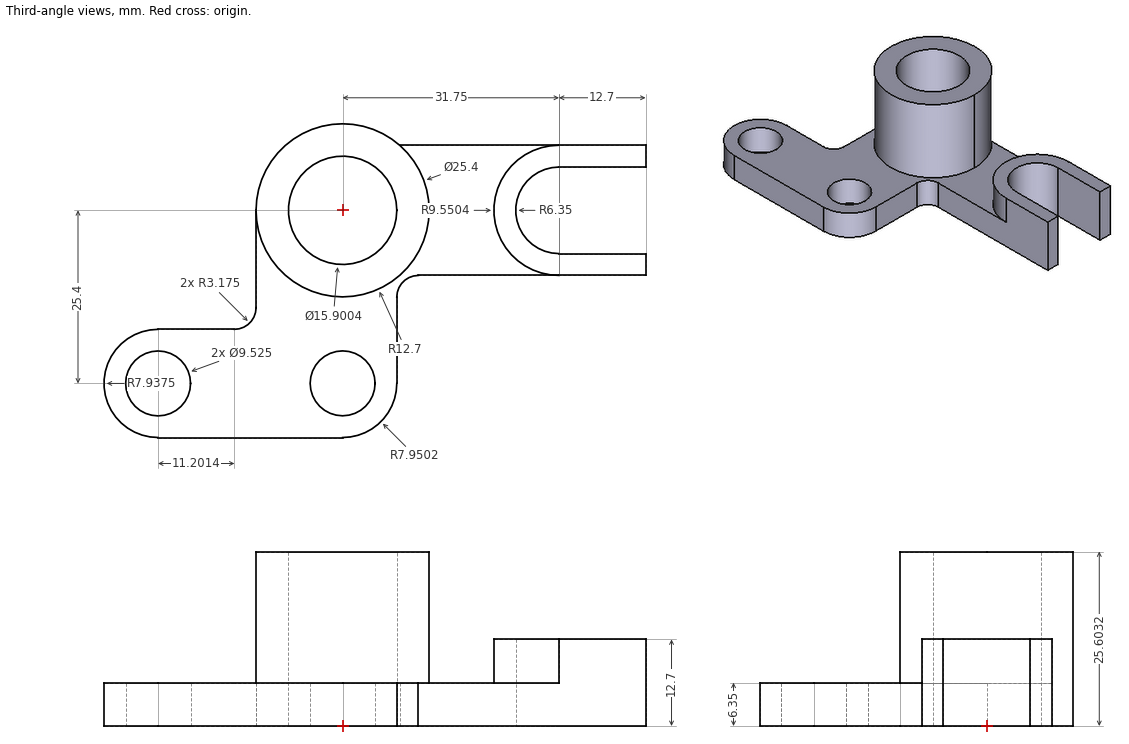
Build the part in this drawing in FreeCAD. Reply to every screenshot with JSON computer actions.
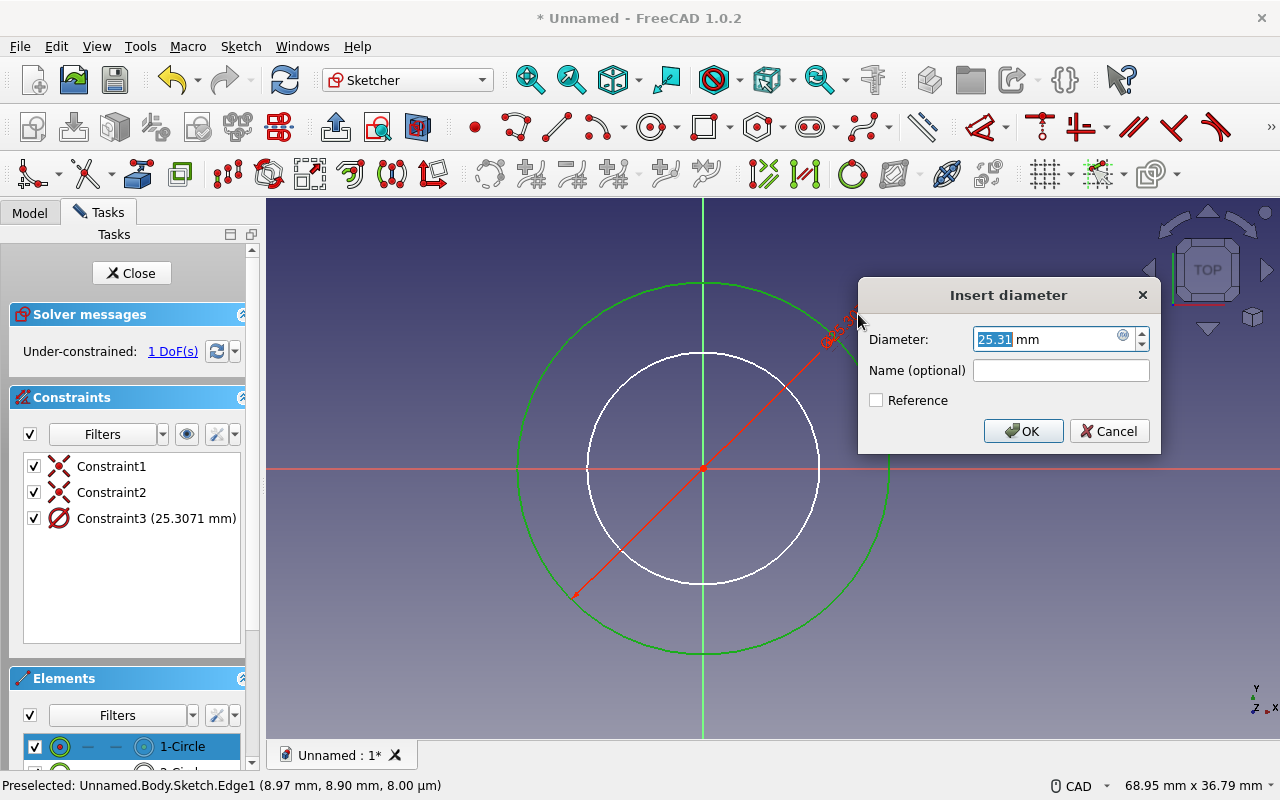
{"action": "type", "text": "25.4"}
{"action": "key", "text": "Return"}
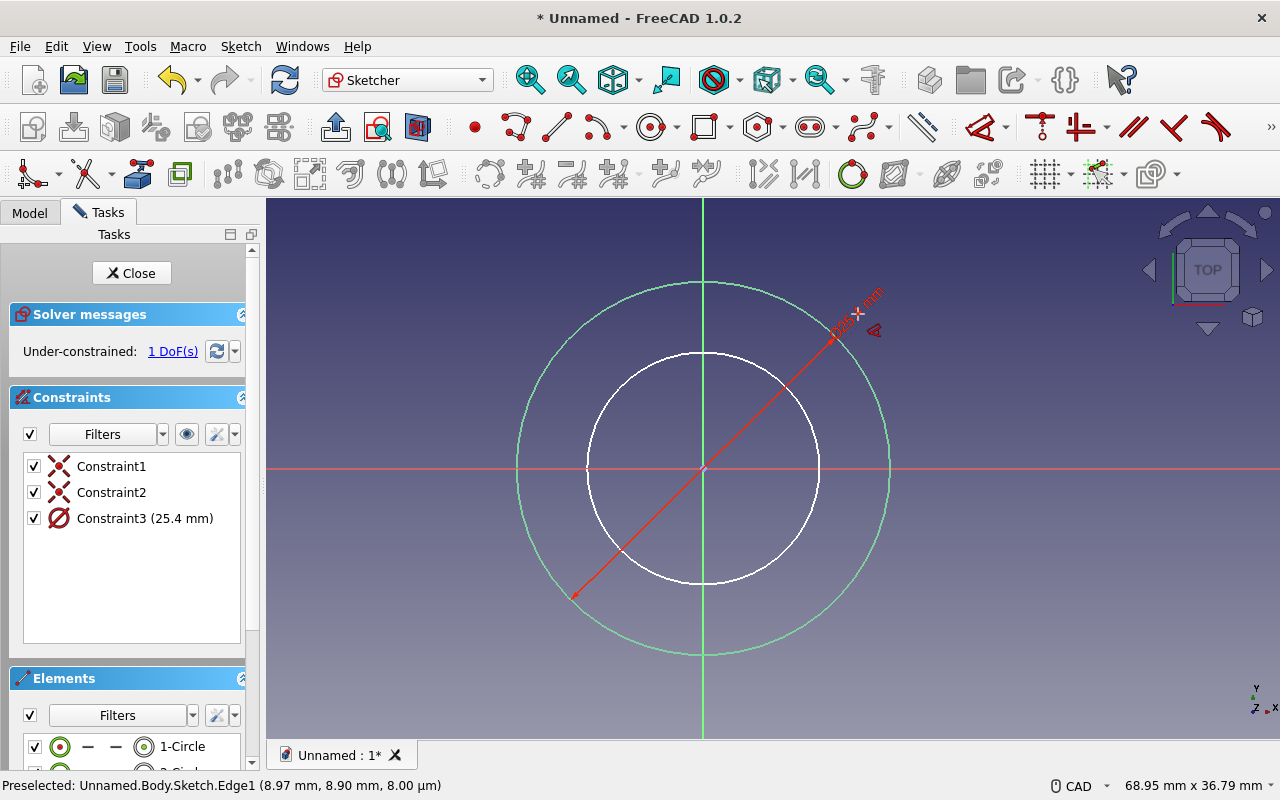
{"action": "left_click", "coordinate": [785, 386]}
{"action": "left_click", "coordinate": [808, 363]}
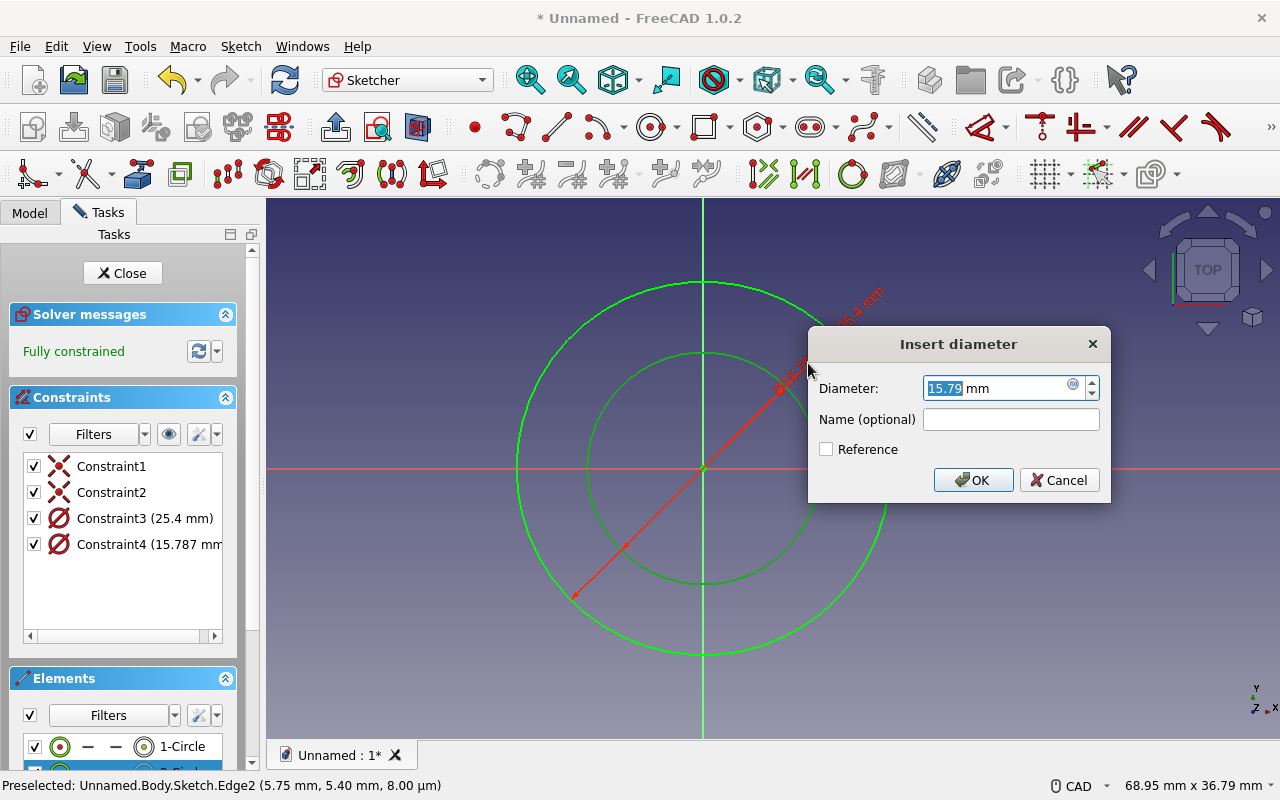
{"action": "type", "text": "15.9004"}
{"action": "key", "text": "Return"}
{"action": "key", "text": "Escape"}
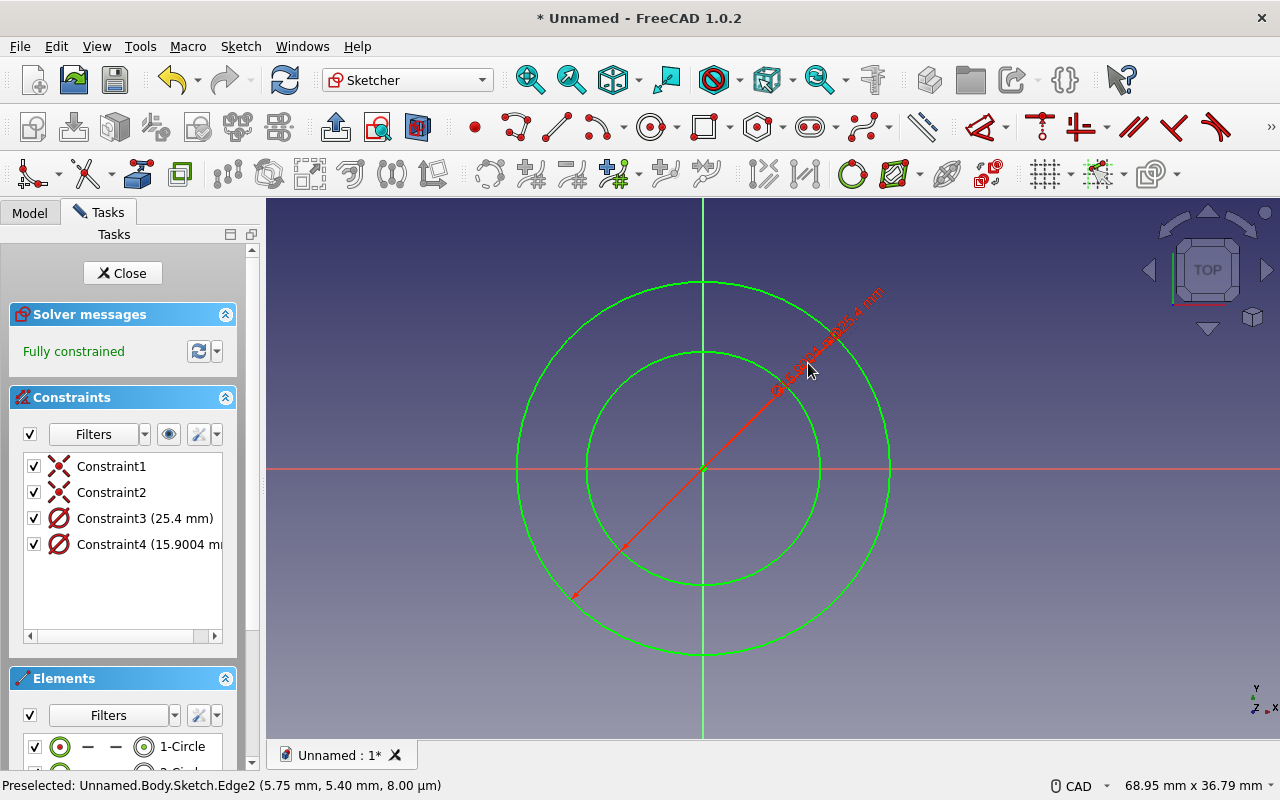
{"action": "left_click", "coordinate": [123, 273]}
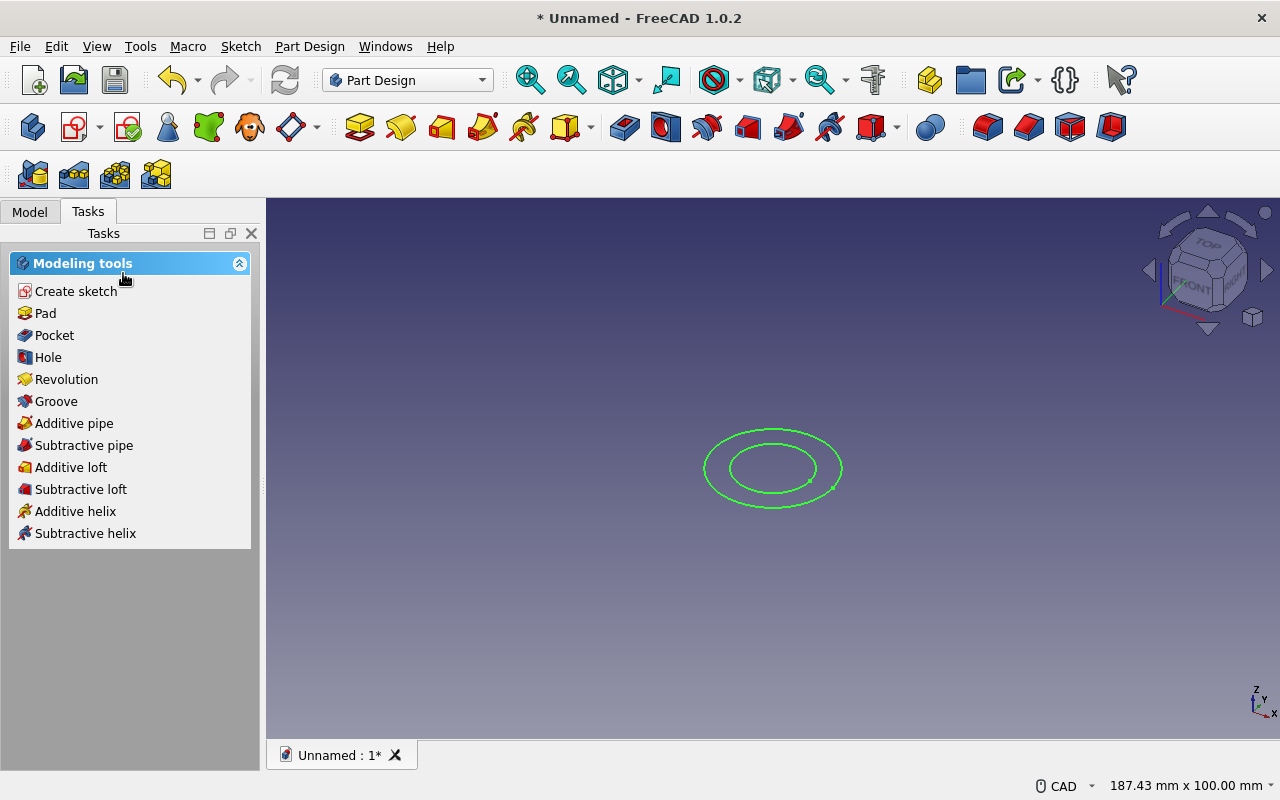
{"action": "left_click", "coordinate": [360, 128]}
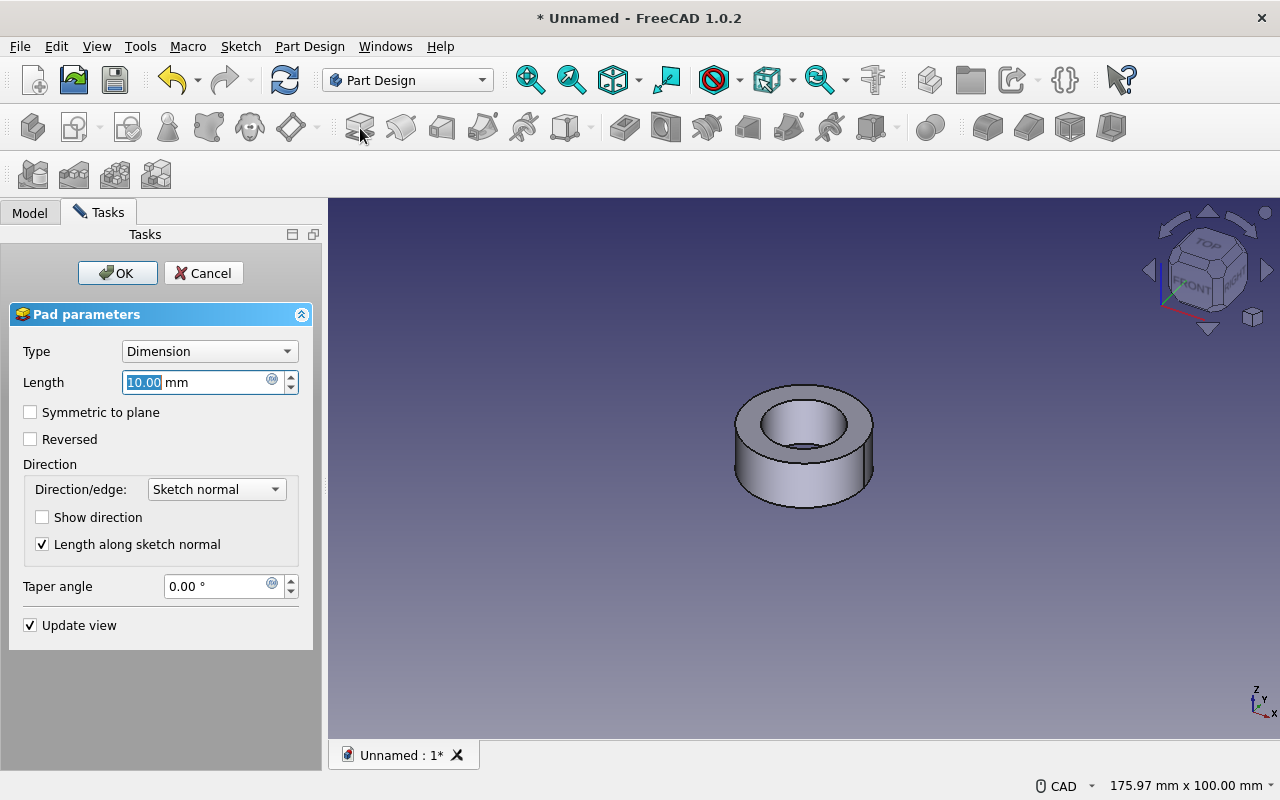
{"action": "type", "text": "25.6032"}
{"action": "key", "text": "Tab"}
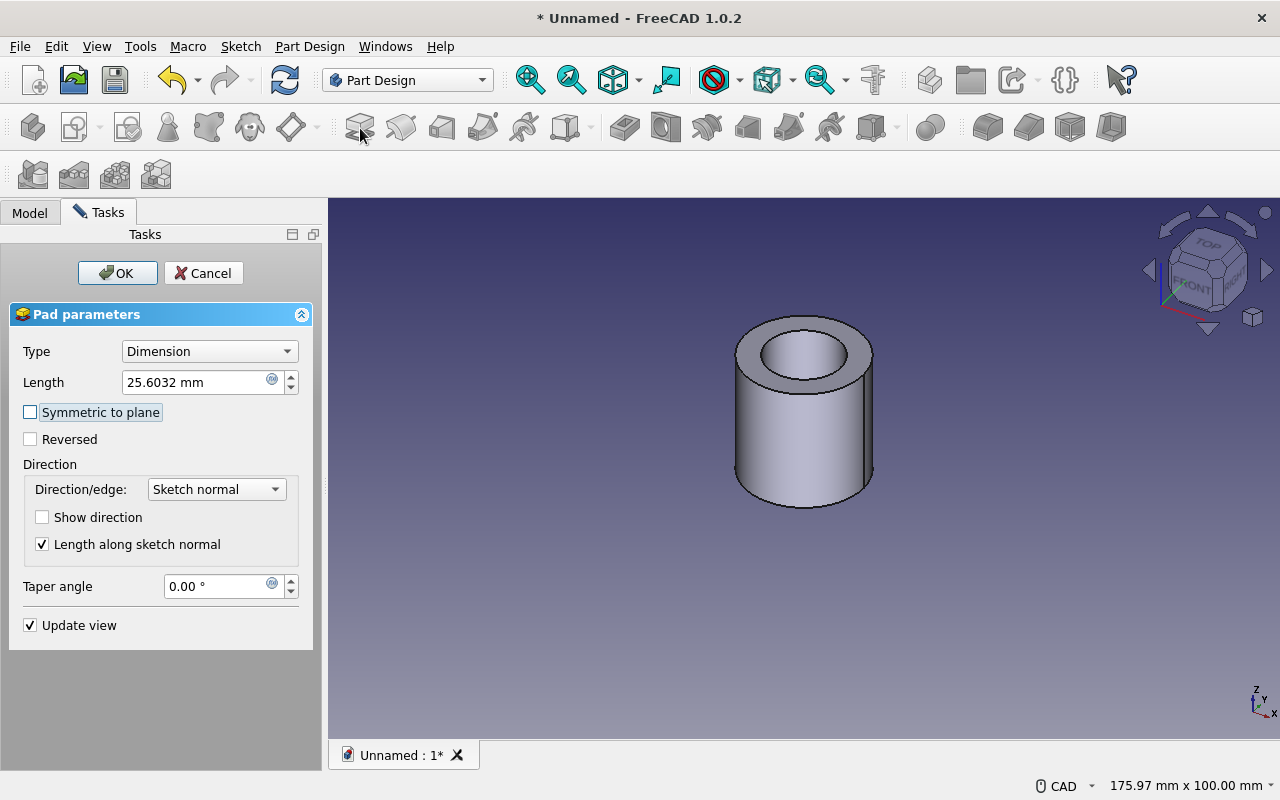
{"action": "left_click", "coordinate": [118, 273]}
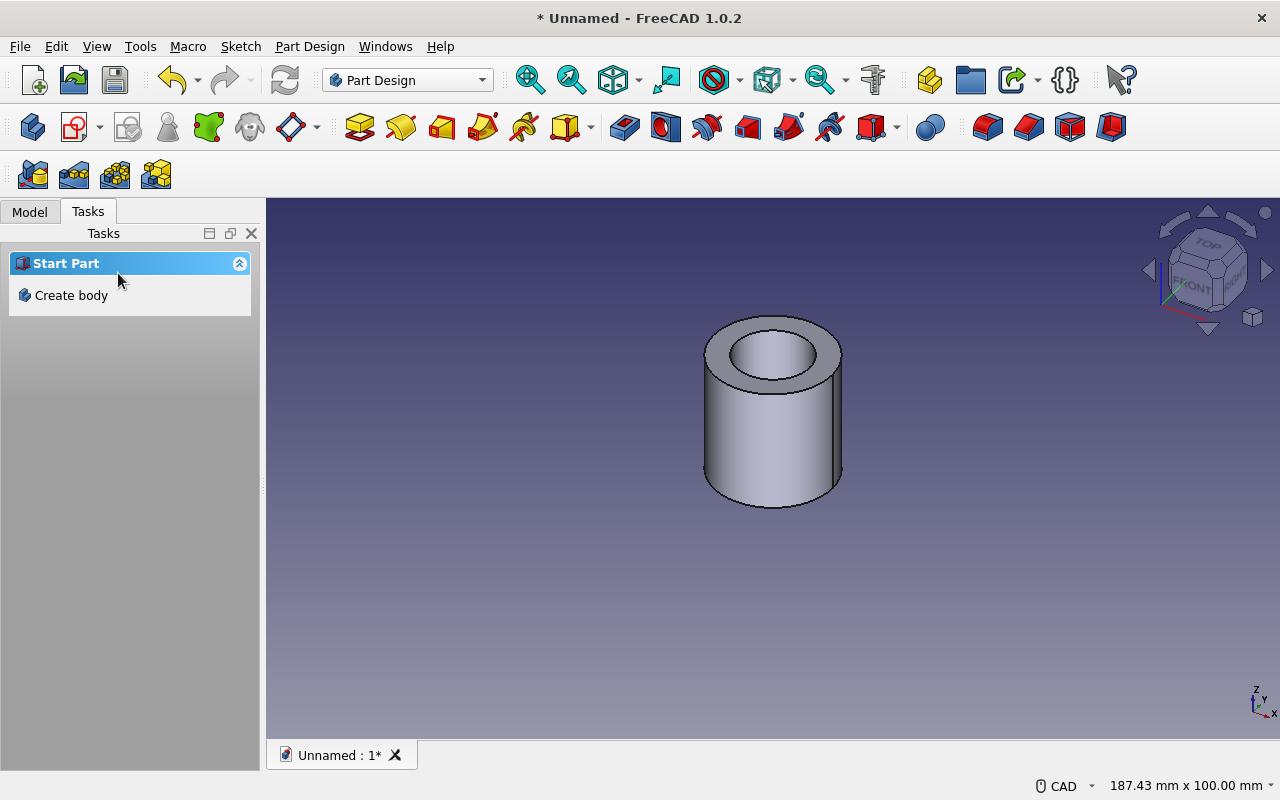
{"action": "left_click", "coordinate": [531, 80]}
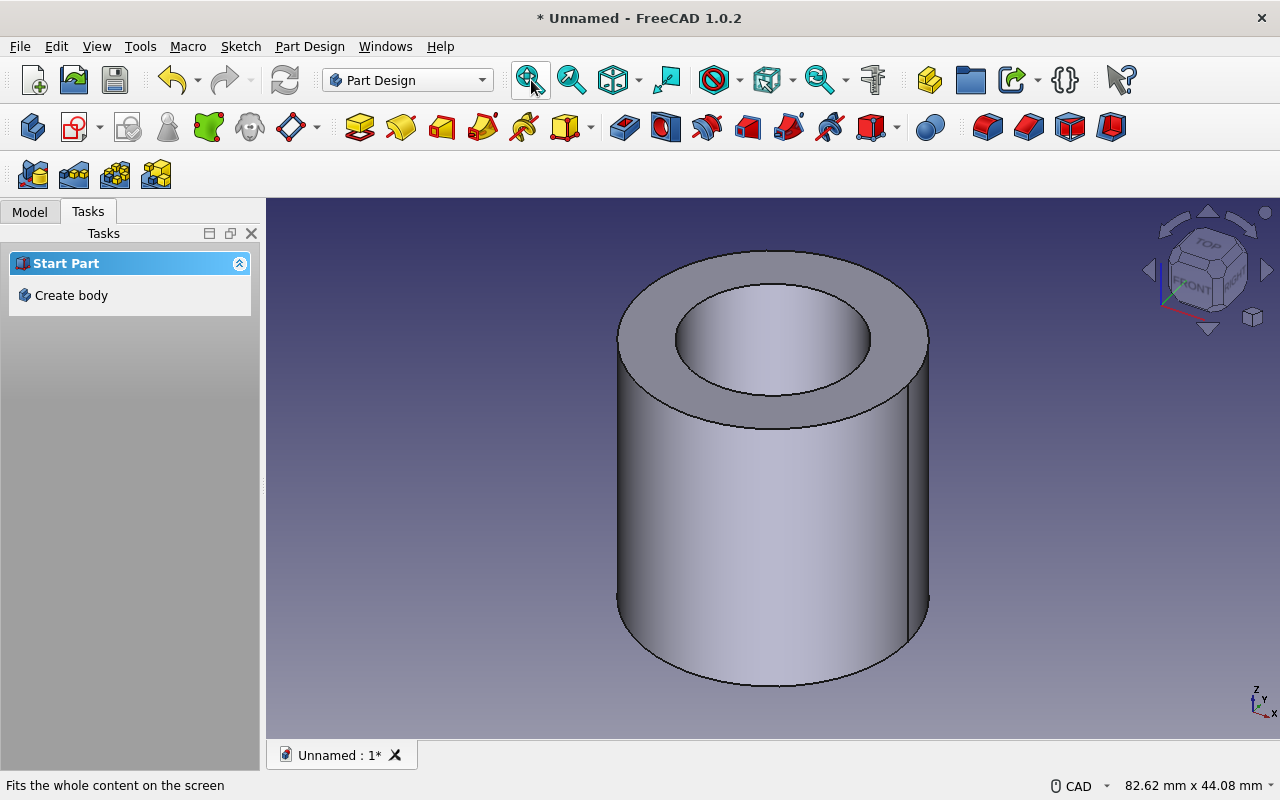
{"action": "left_click", "coordinate": [33, 128]}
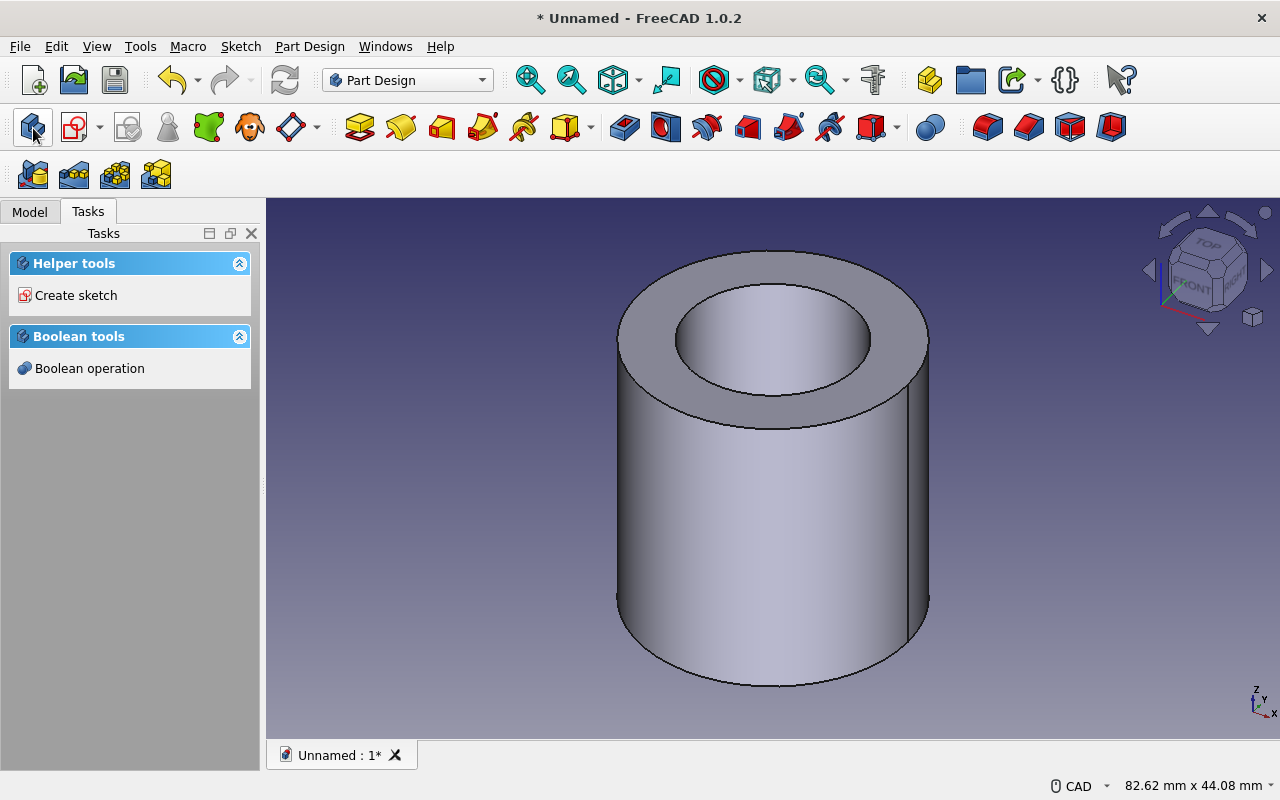
{"action": "left_click", "coordinate": [306, 699]}